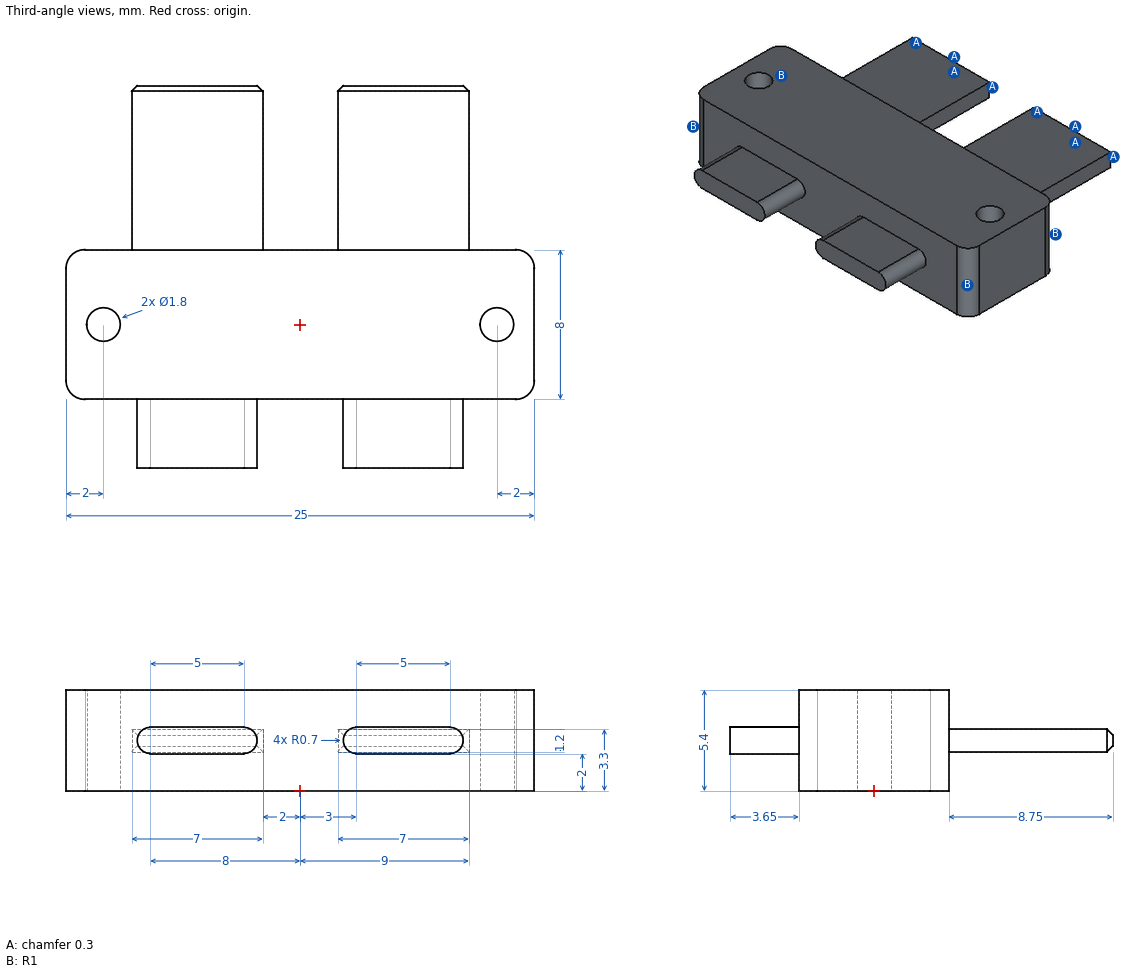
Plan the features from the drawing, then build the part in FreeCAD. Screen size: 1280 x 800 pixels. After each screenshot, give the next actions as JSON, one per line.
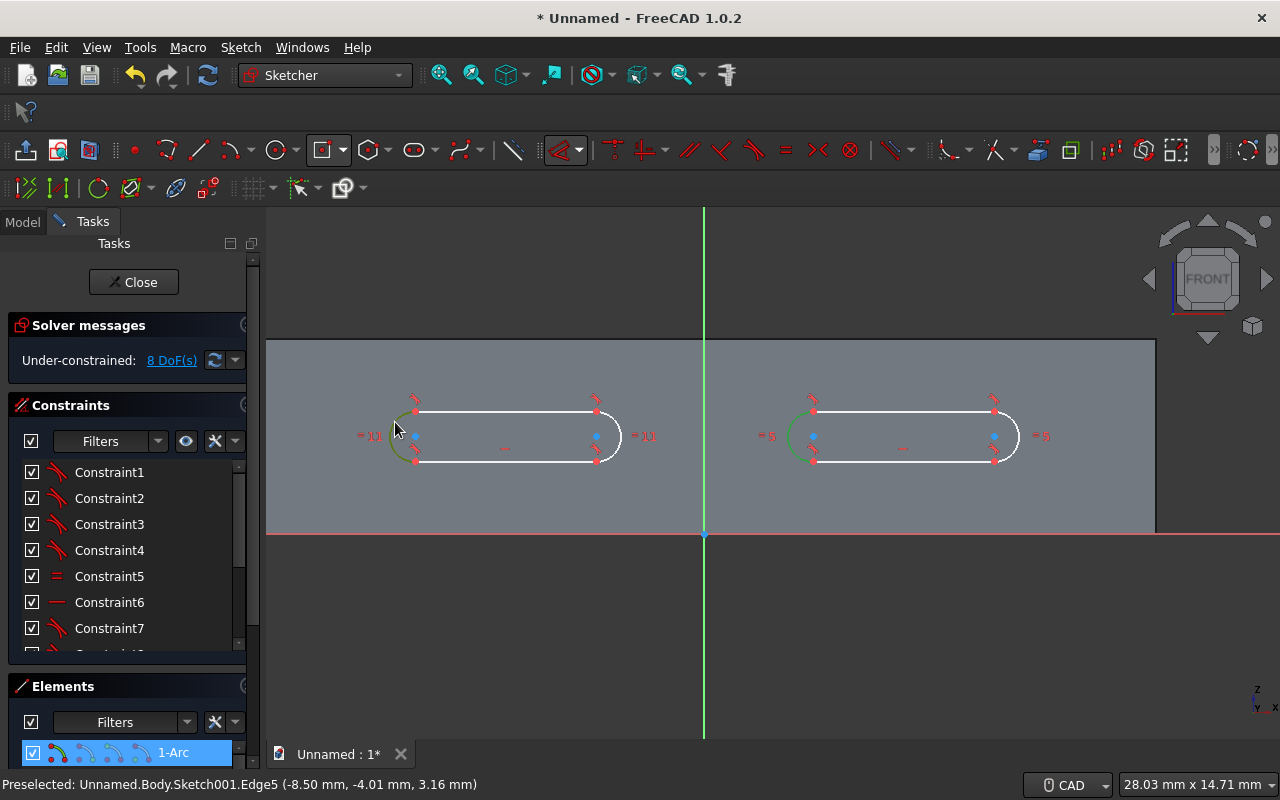
{"action": "left_click", "coordinate": [786, 150]}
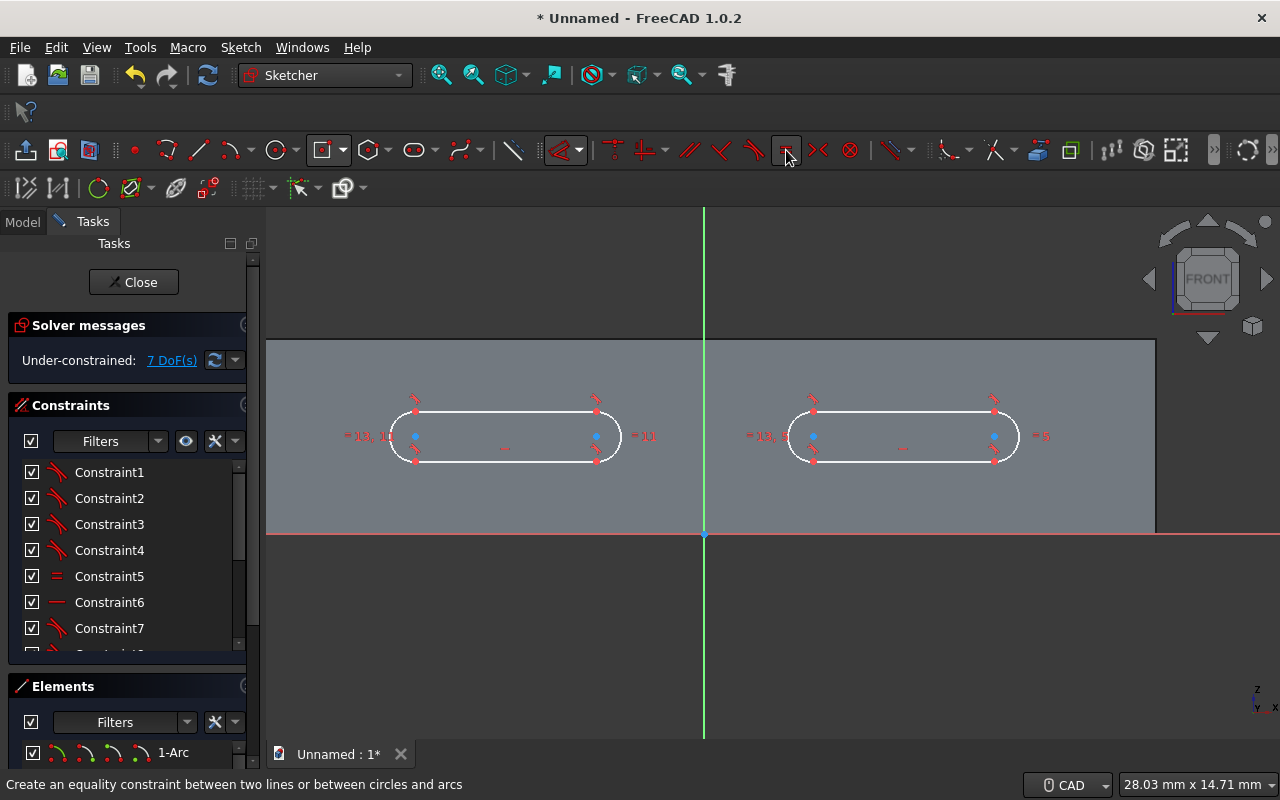
{"action": "scroll", "coordinate": [793, 422], "scroll_direction": "up", "scroll_amount": 3}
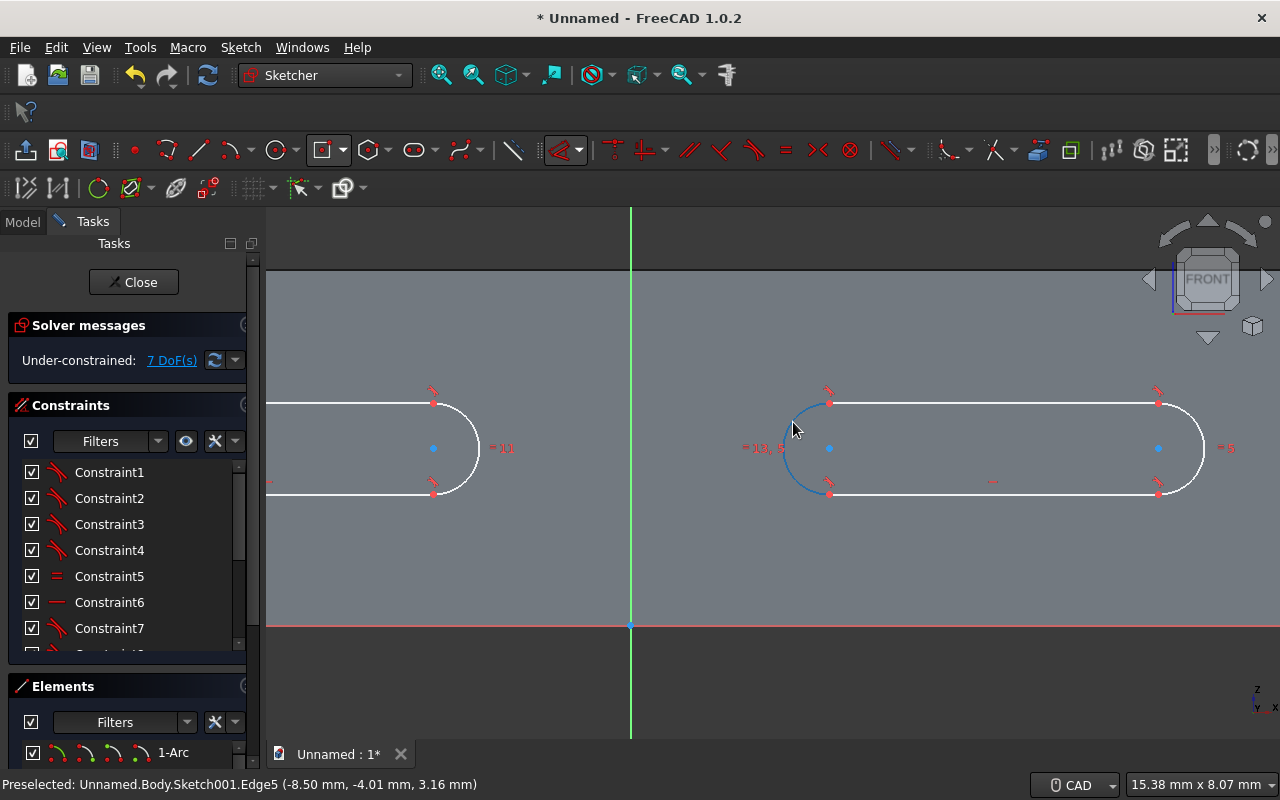
{"action": "left_click", "coordinate": [792, 422]}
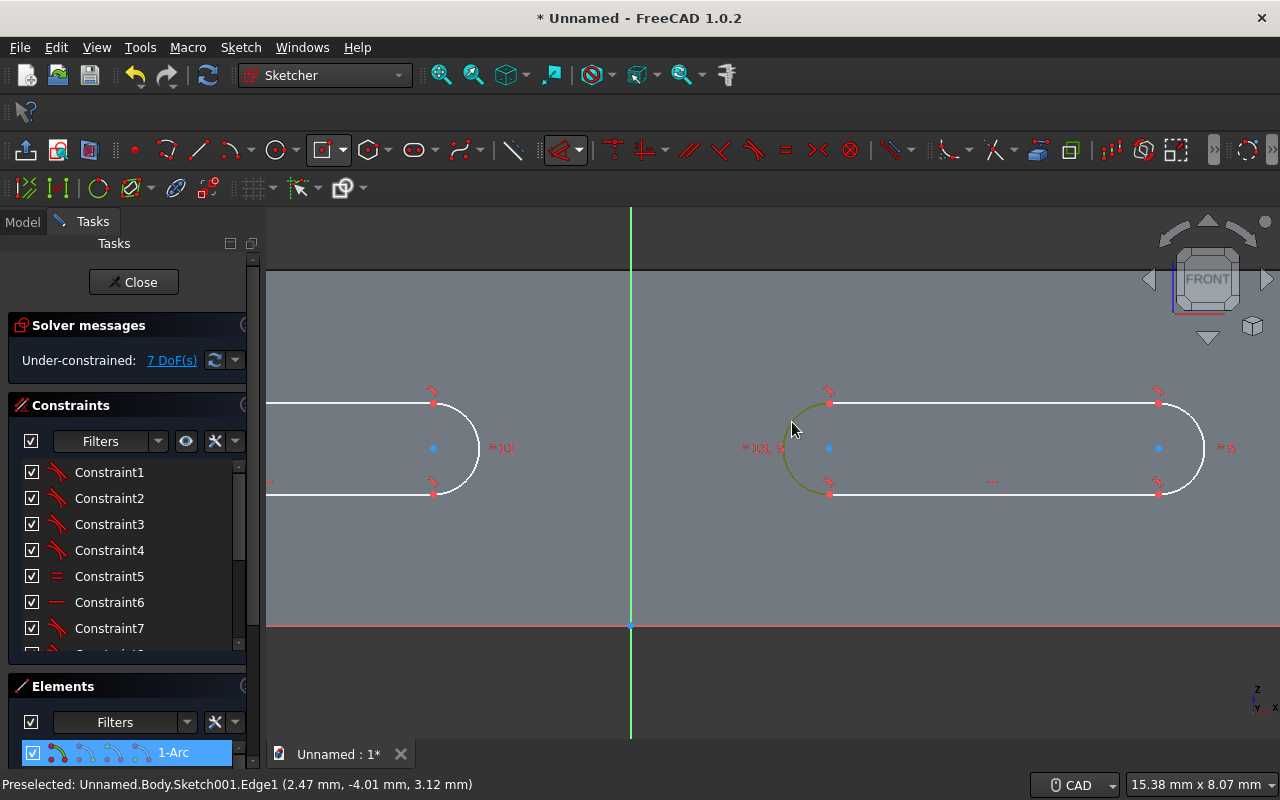
{"action": "key", "text": "k r"}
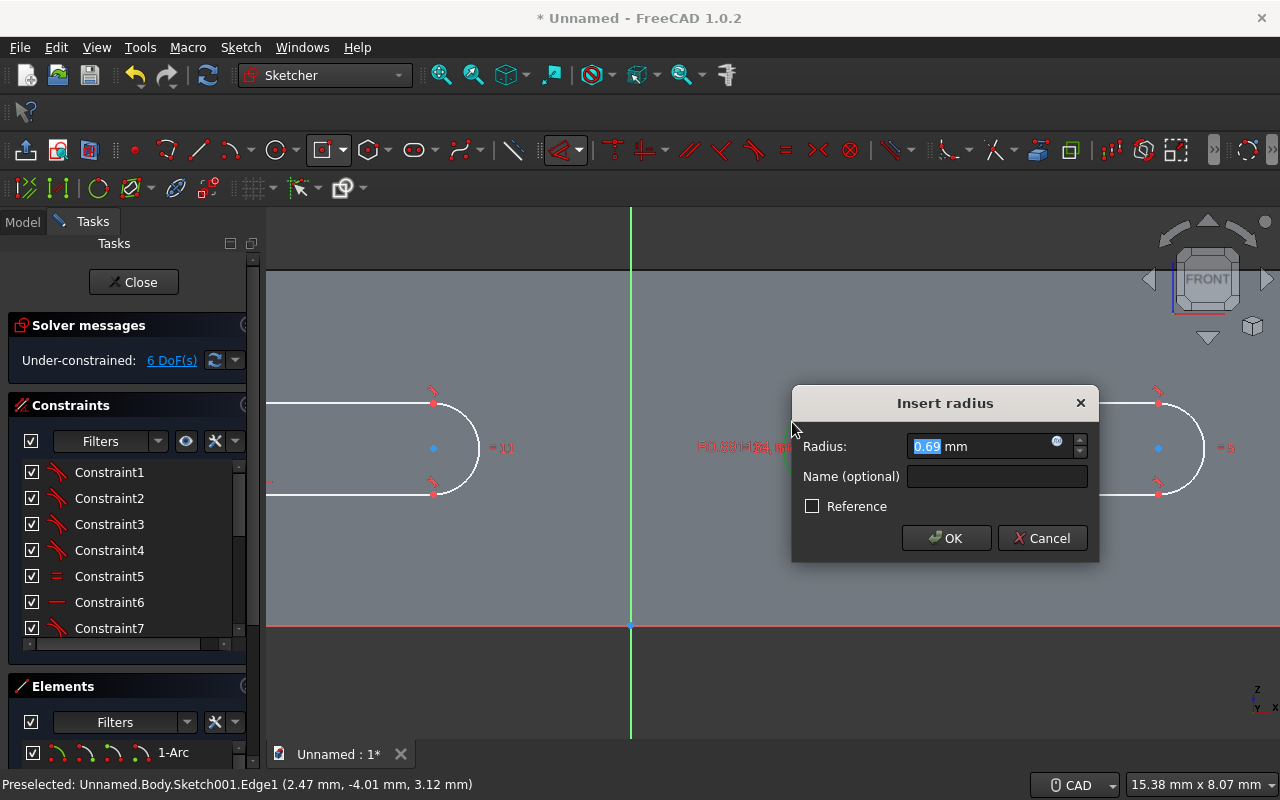
{"action": "type", "text": "0.7"}
{"action": "key", "text": "Return"}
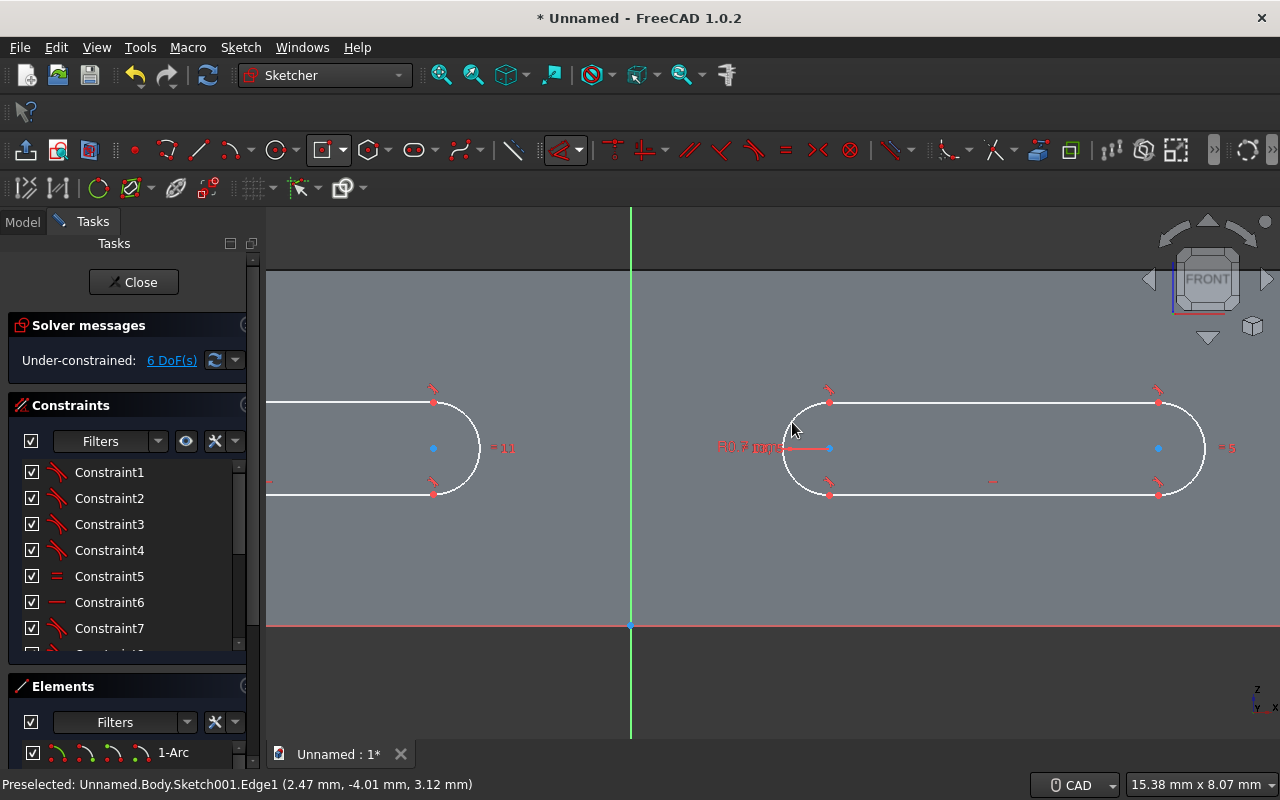
{"action": "left_click", "coordinate": [928, 403]}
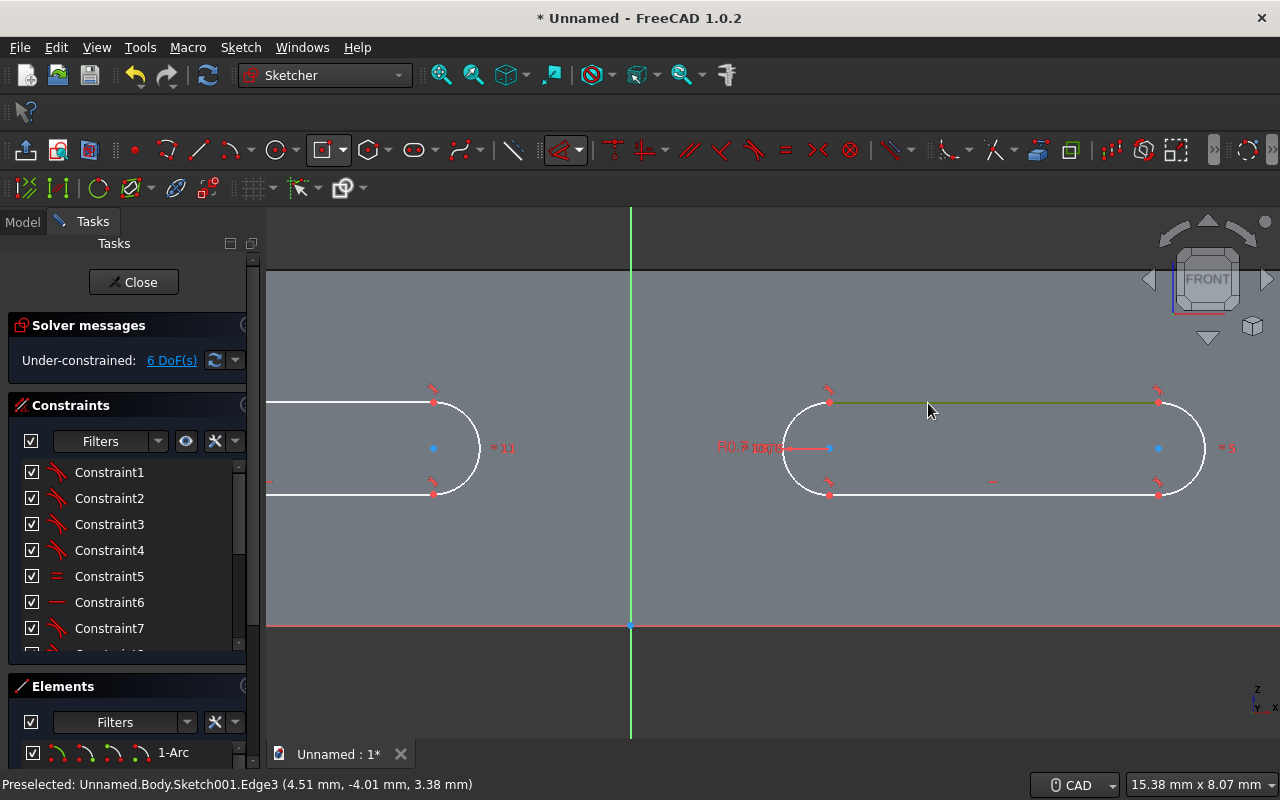
{"action": "key", "text": "l"}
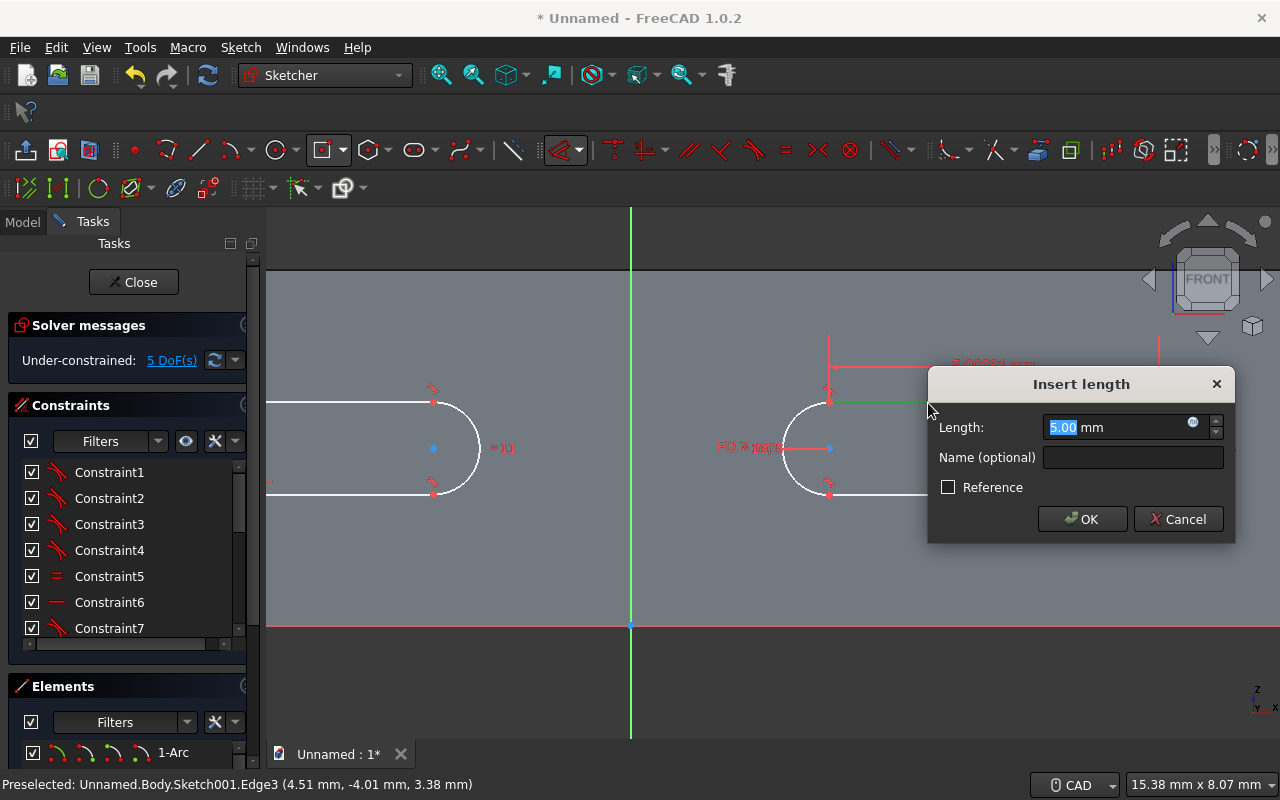
{"action": "type", "text": "5"}
{"action": "key", "text": "Return"}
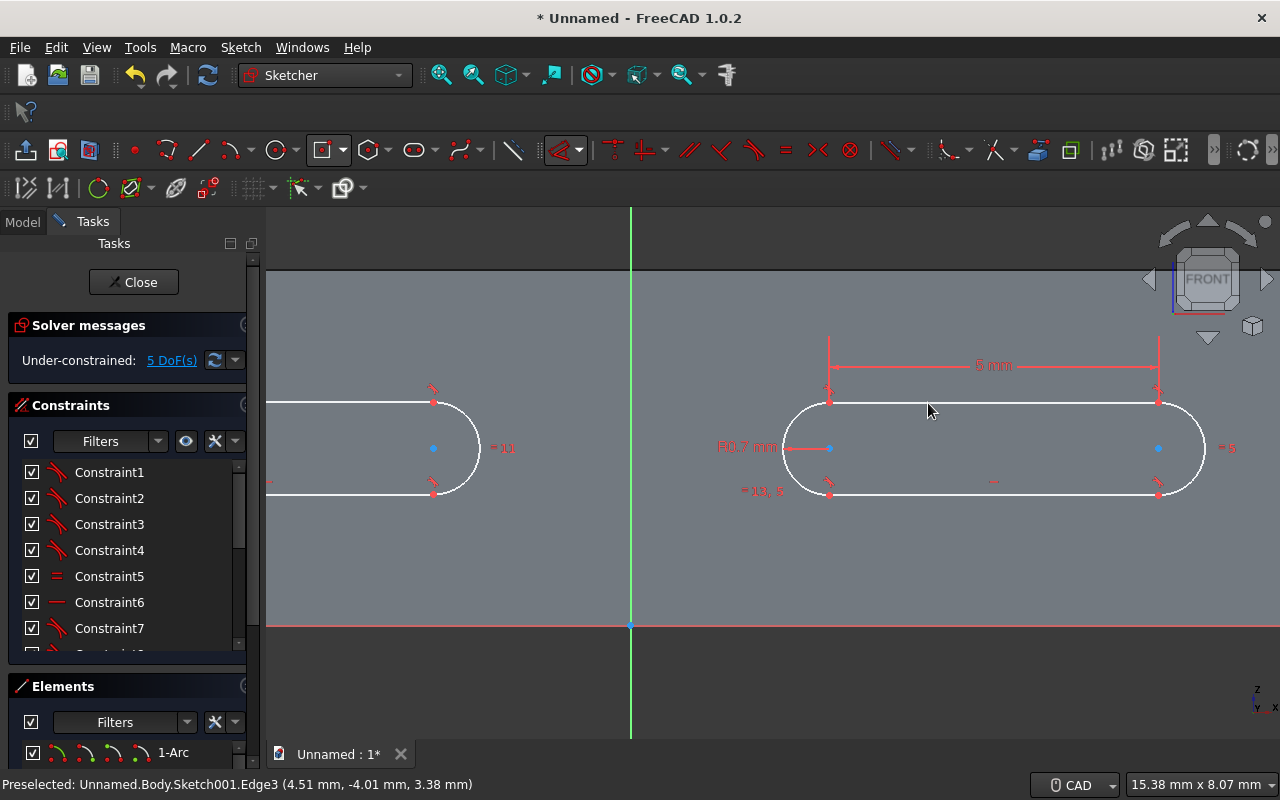
{"action": "left_click", "coordinate": [335, 402]}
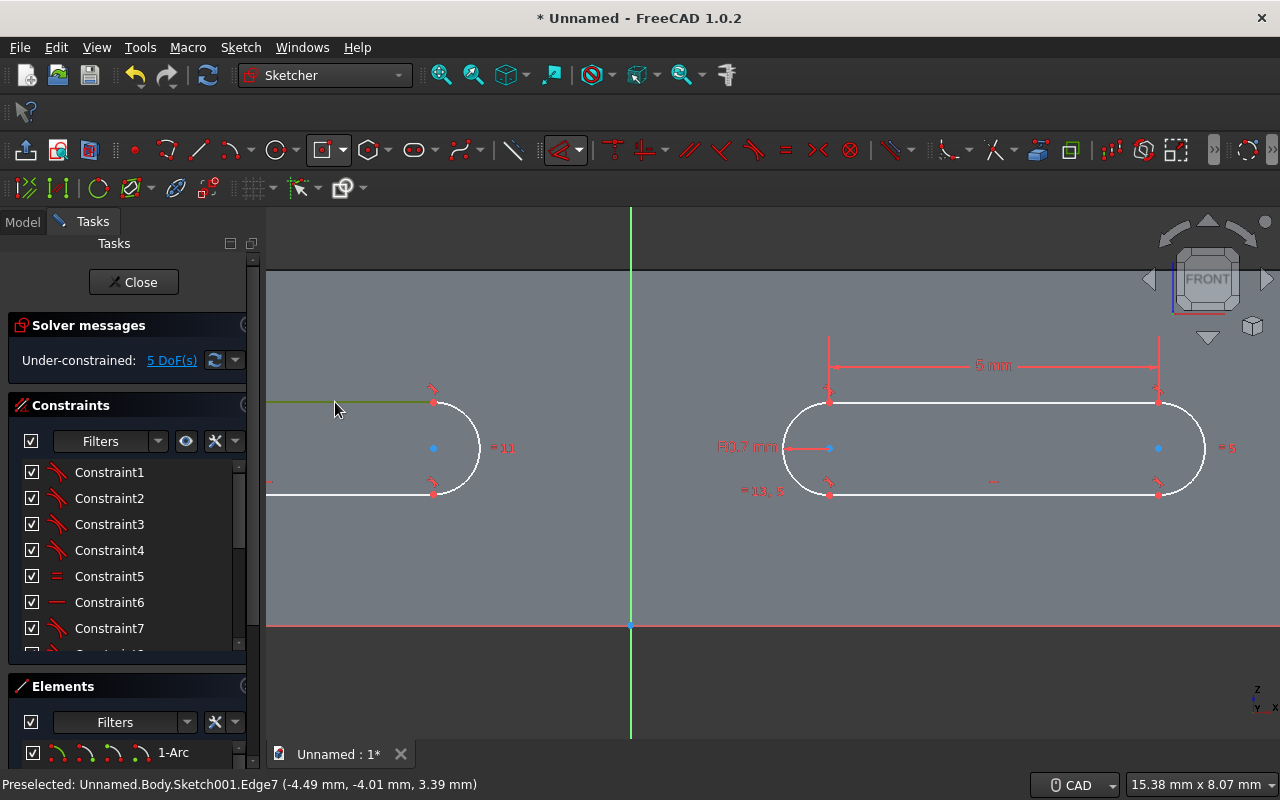
{"action": "left_click", "coordinate": [582, 150]}